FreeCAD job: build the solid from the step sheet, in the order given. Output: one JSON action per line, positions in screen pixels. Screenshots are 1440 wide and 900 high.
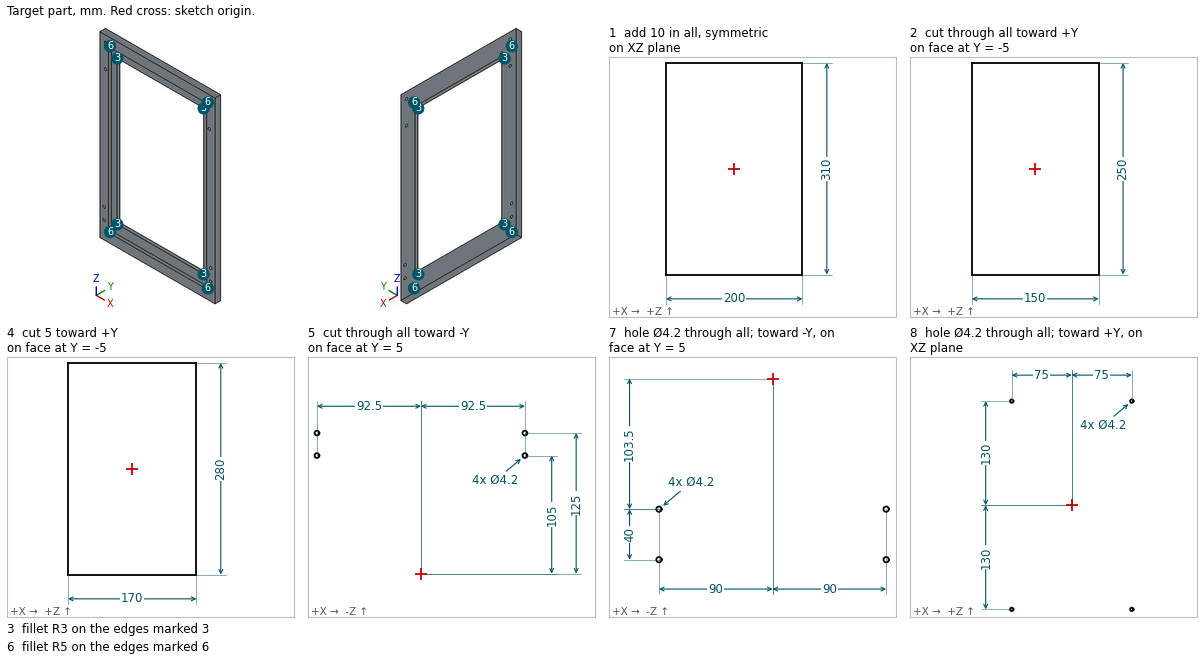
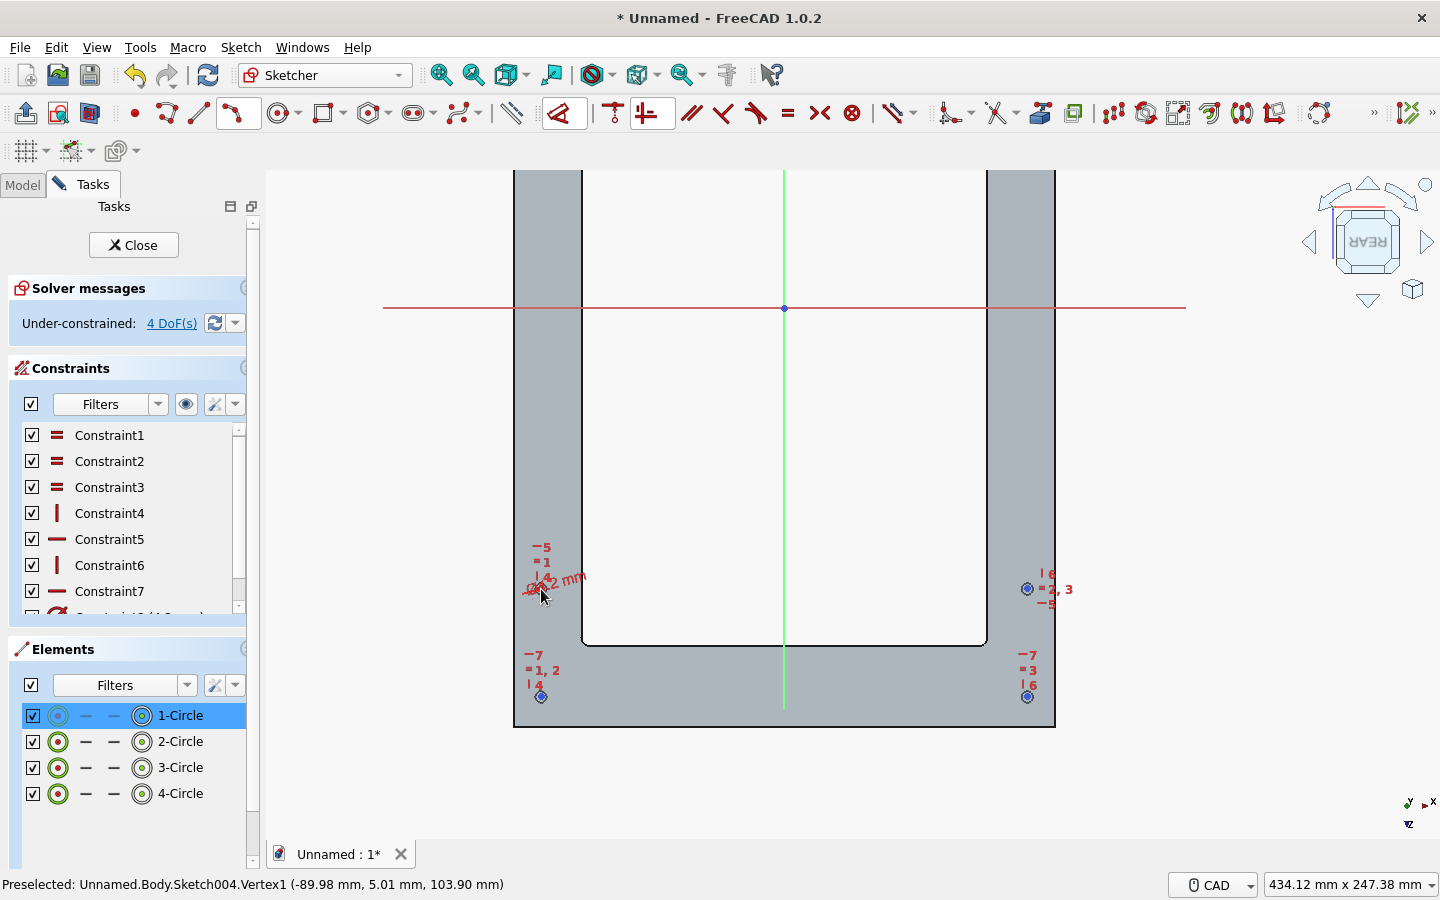
{"action": "key", "text": "l"}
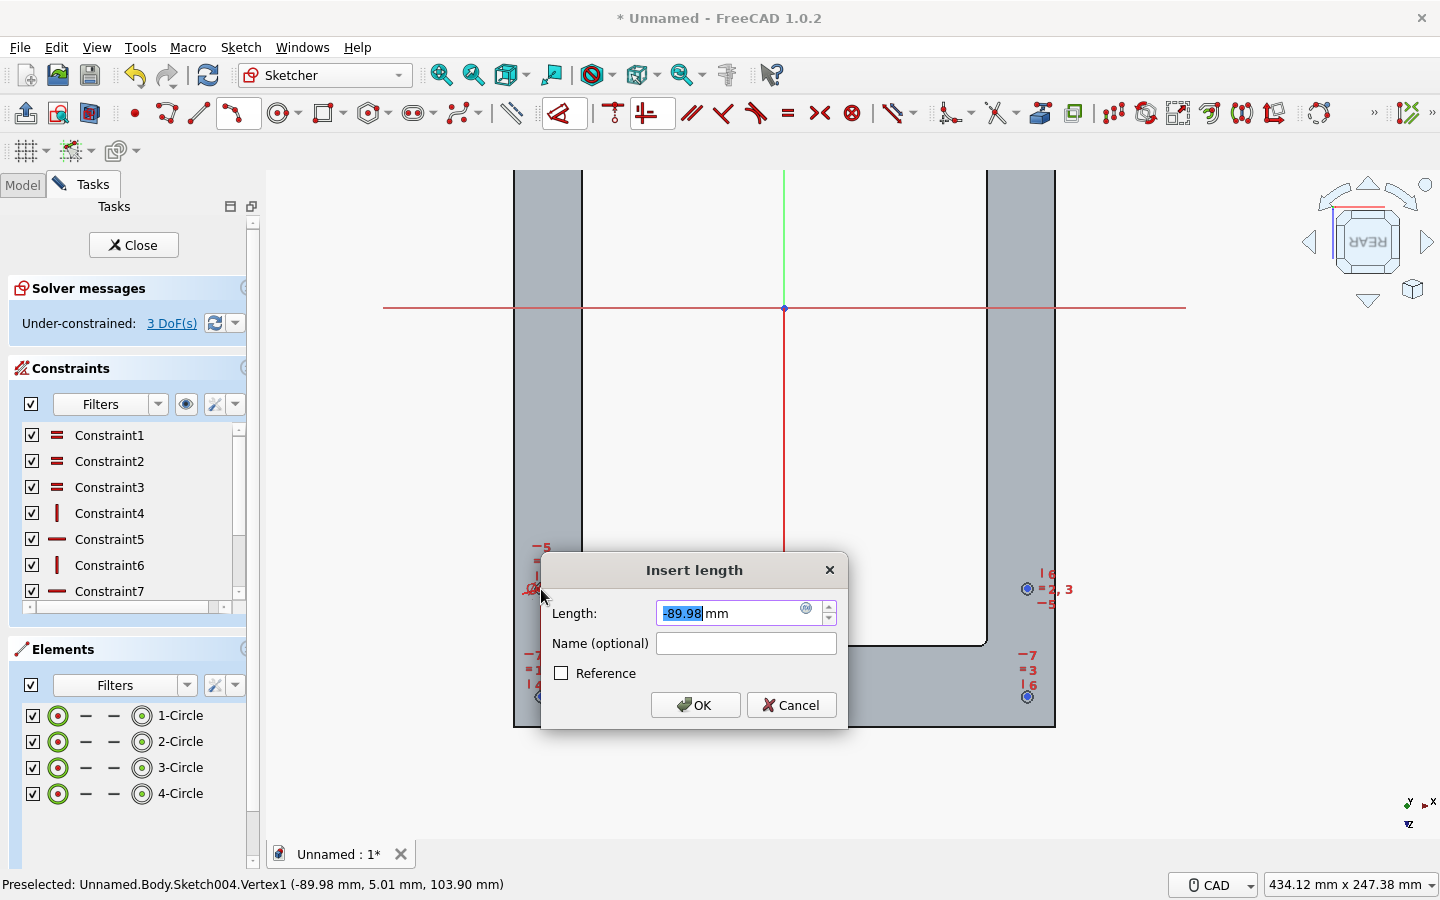
{"action": "type", "text": "-90"}
{"action": "key", "text": "Return"}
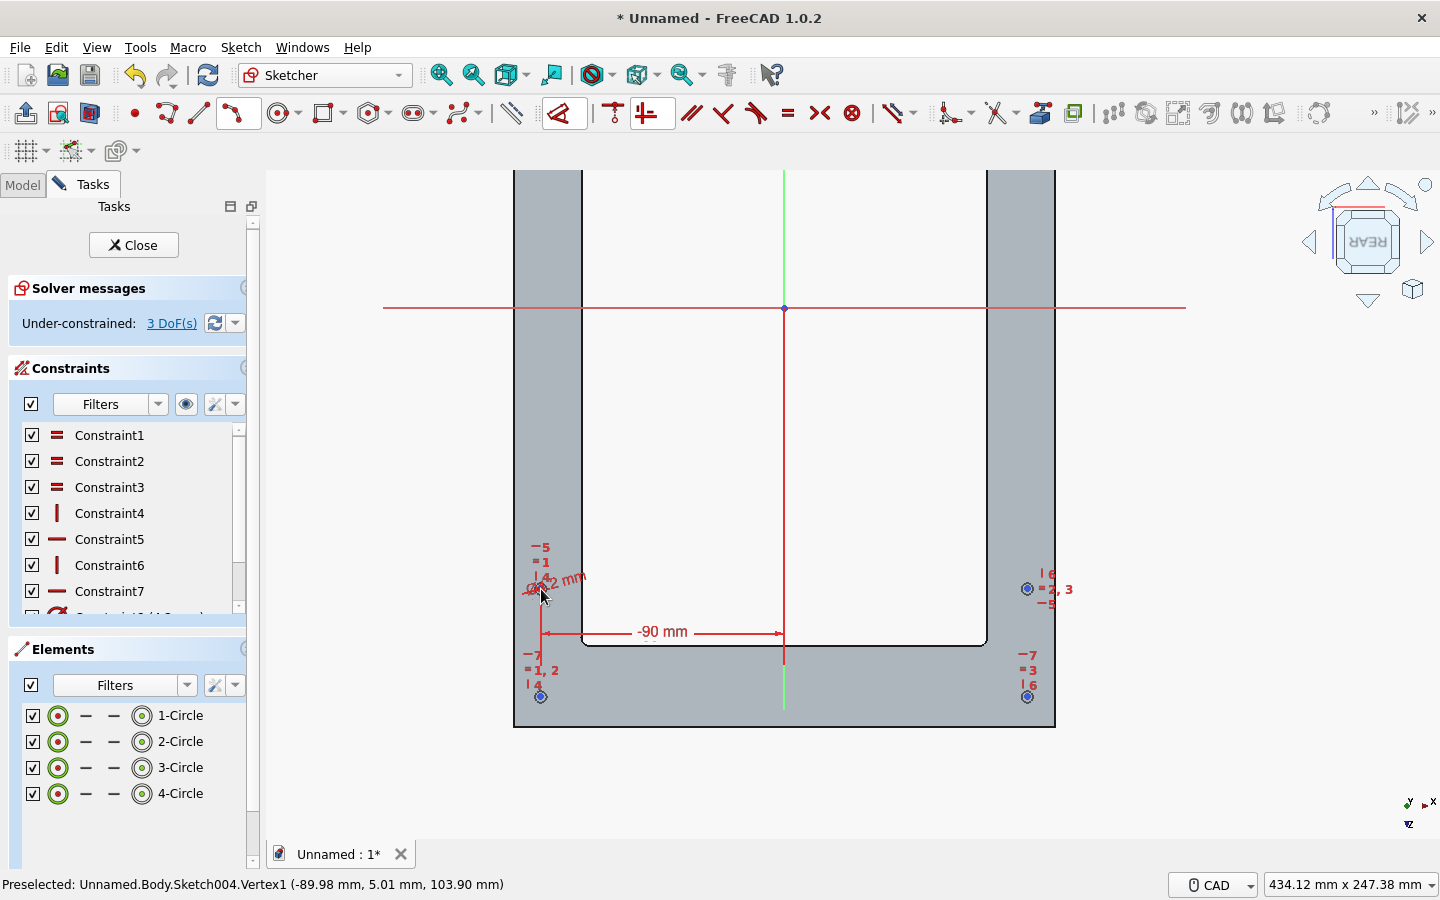
{"action": "left_click", "coordinate": [1027, 589]}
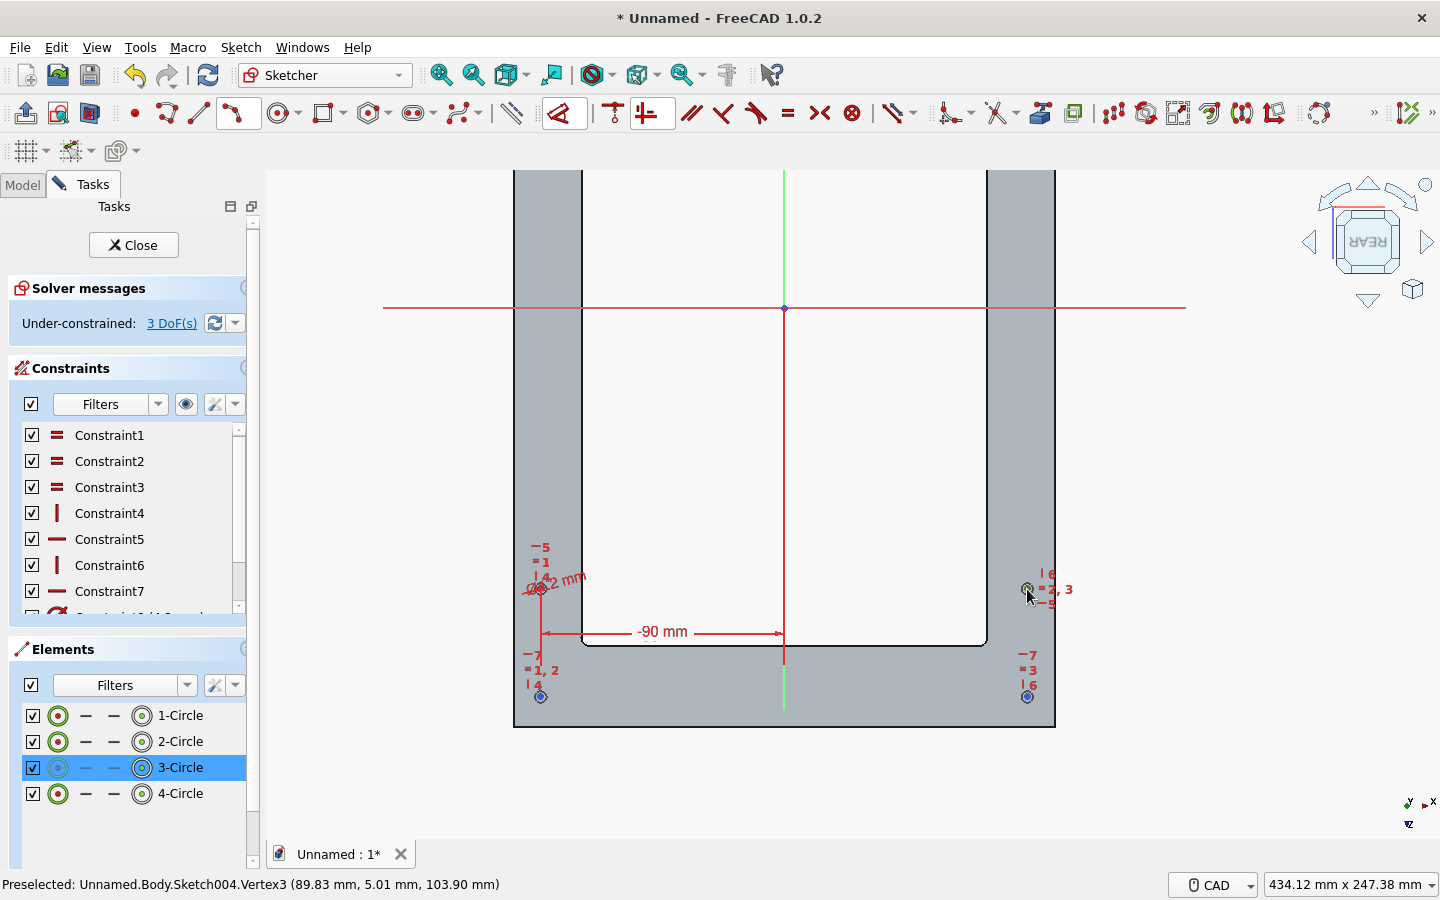
{"action": "left_click", "coordinate": [582, 114]}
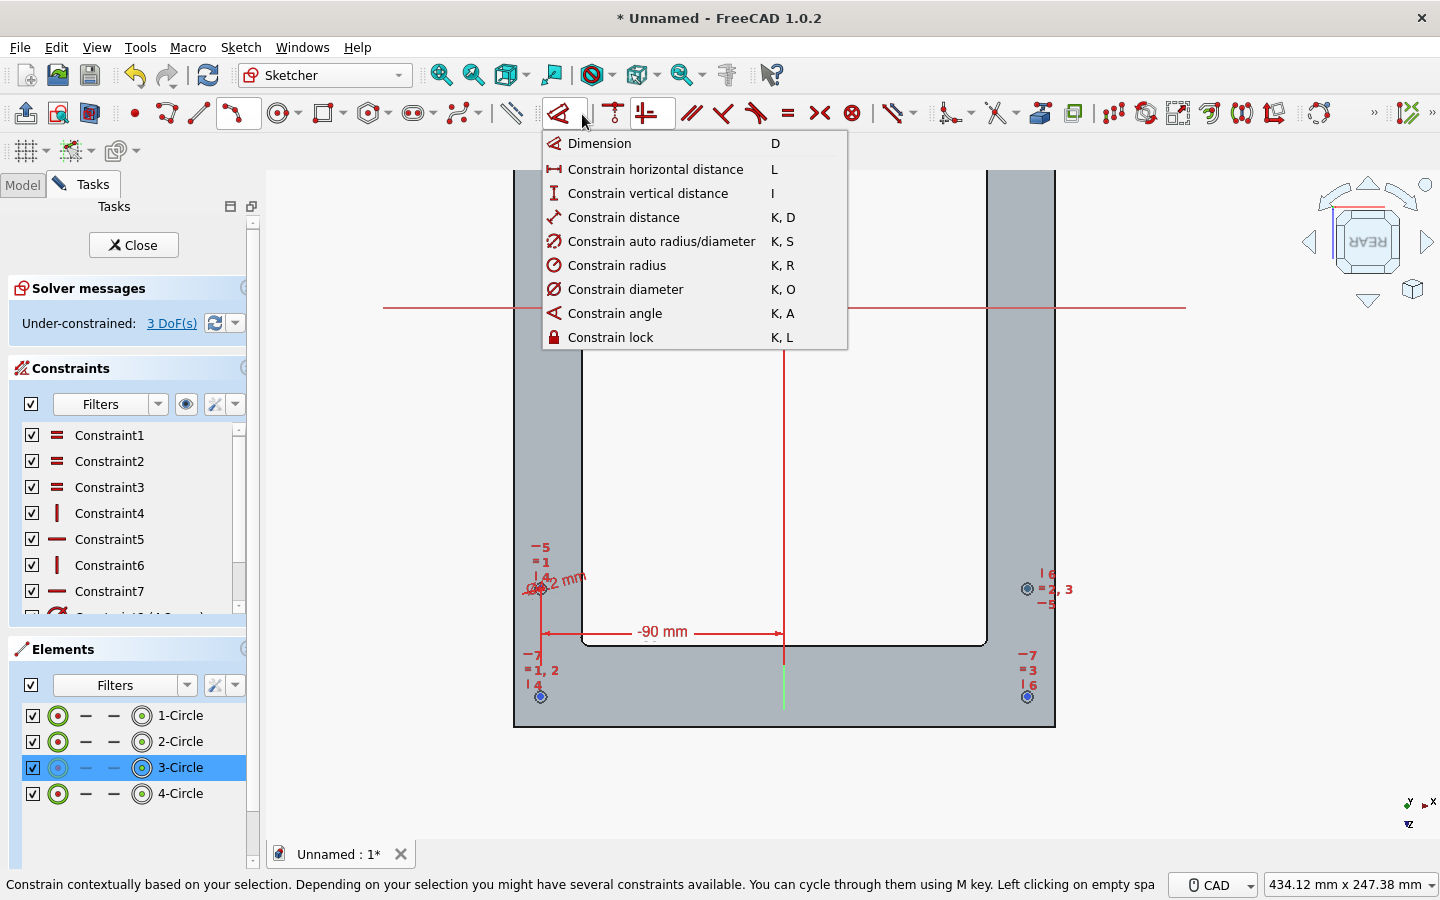
{"action": "left_click", "coordinate": [695, 169]}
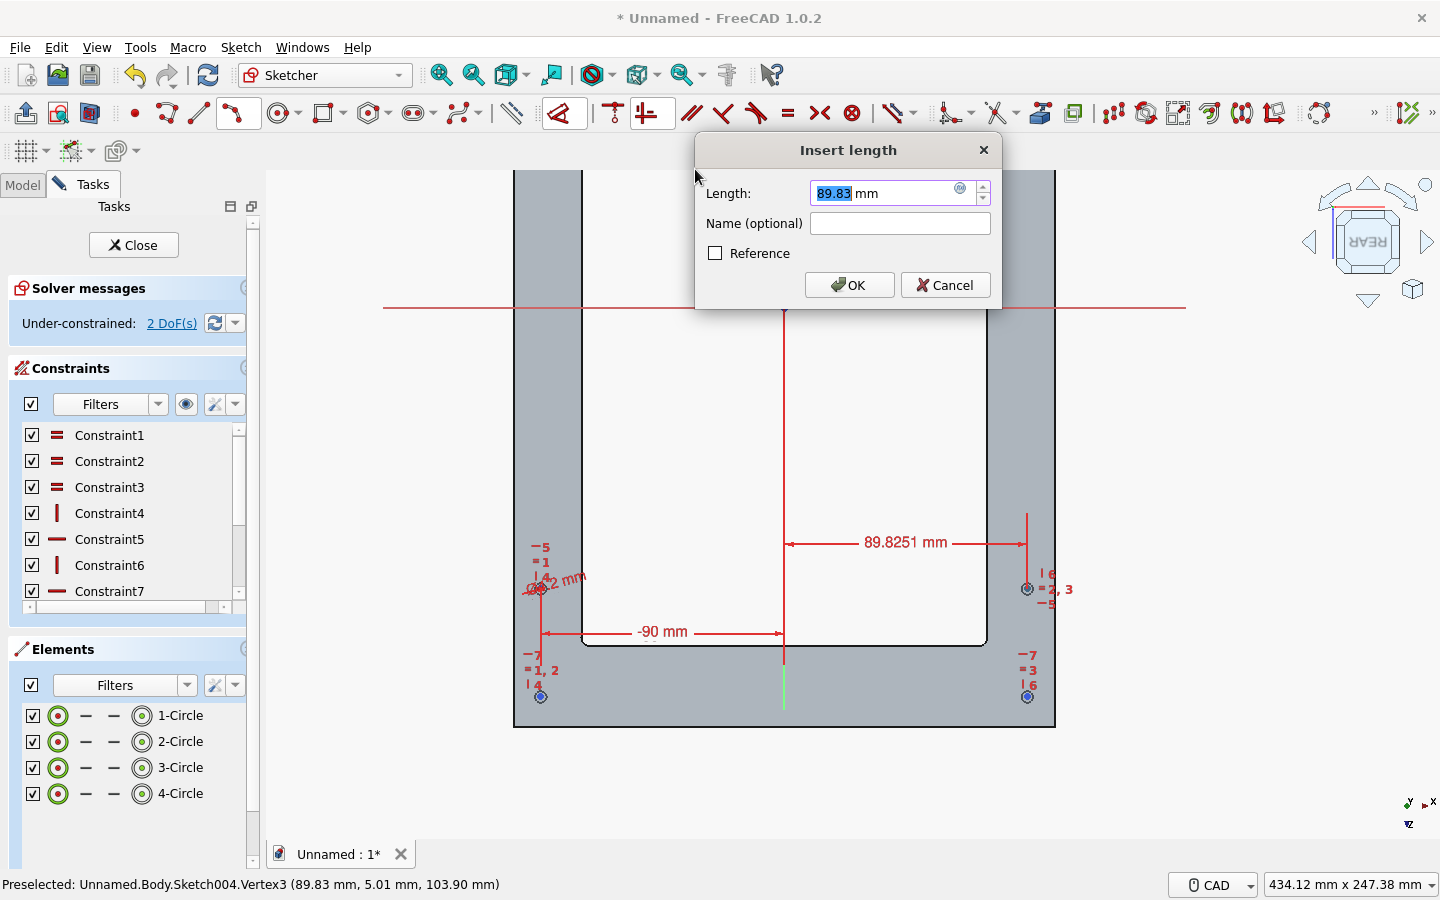
{"action": "type", "text": "90"}
{"action": "key", "text": "Return"}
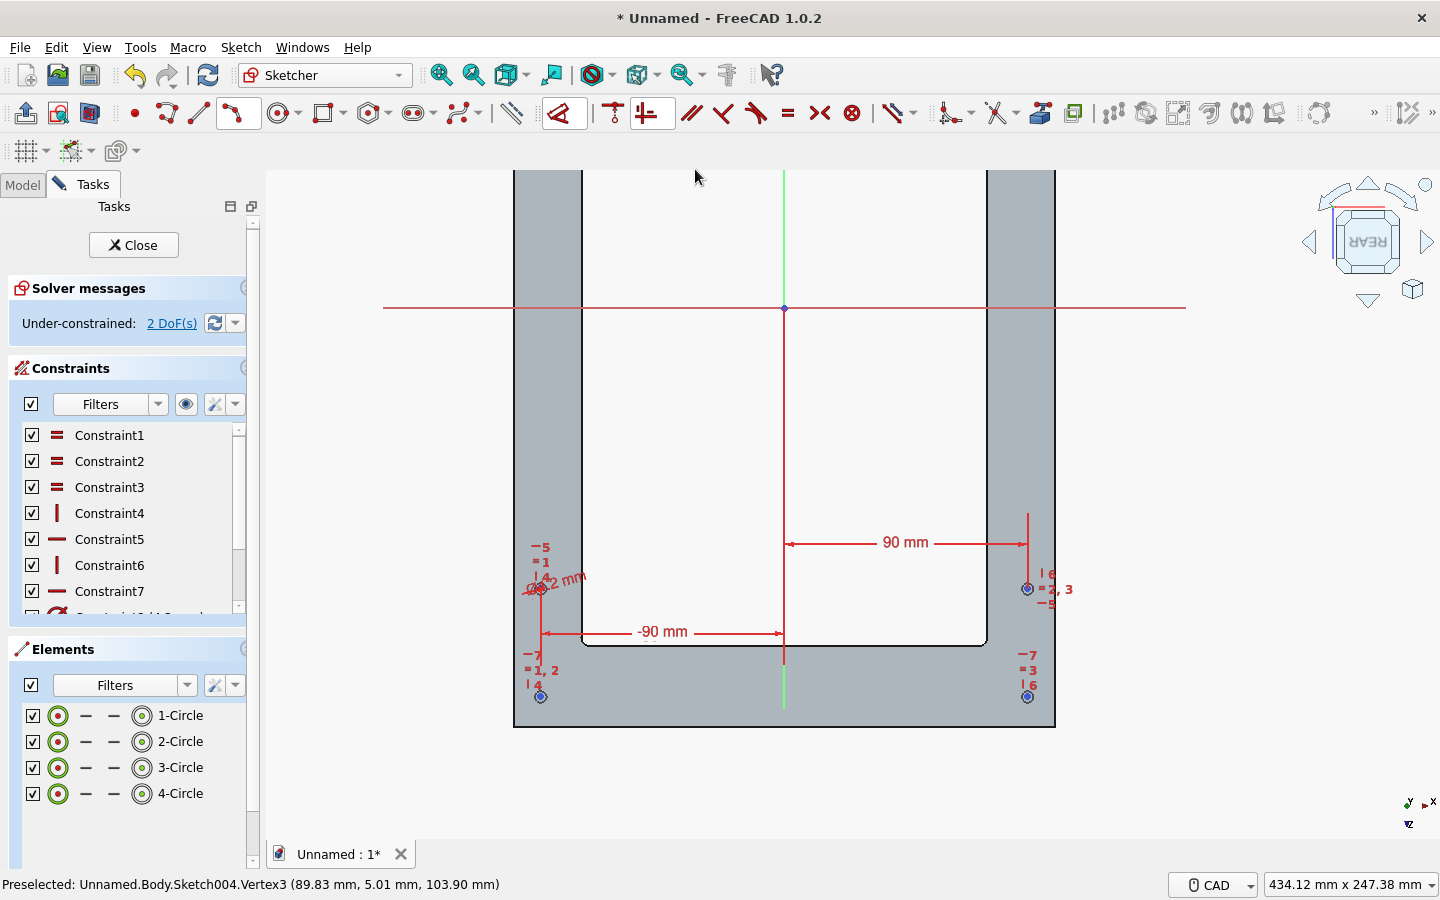
{"action": "left_click", "coordinate": [541, 589]}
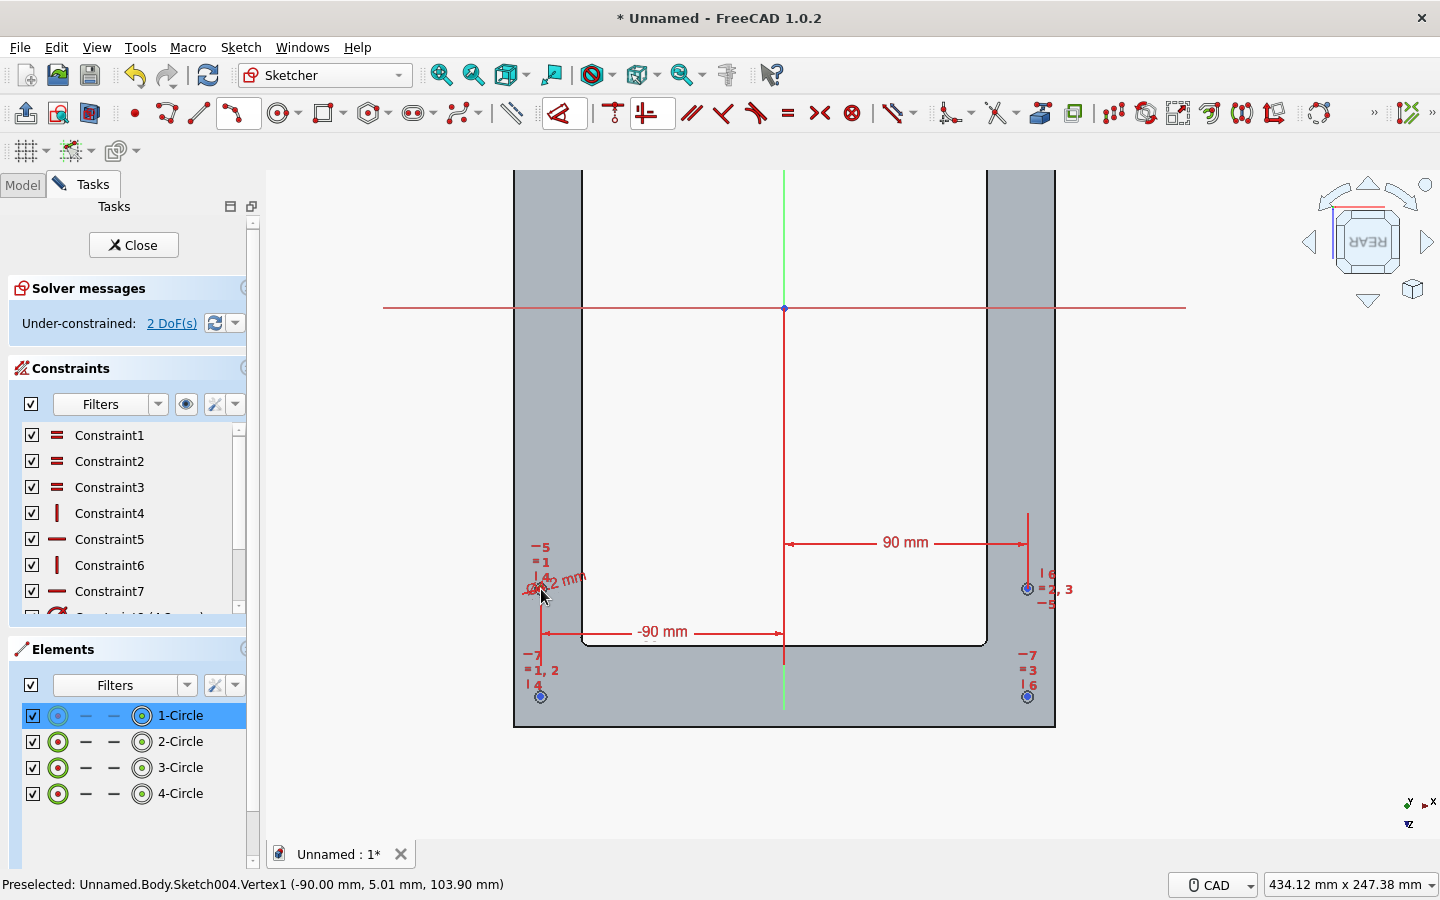
{"action": "left_click", "coordinate": [541, 697]}